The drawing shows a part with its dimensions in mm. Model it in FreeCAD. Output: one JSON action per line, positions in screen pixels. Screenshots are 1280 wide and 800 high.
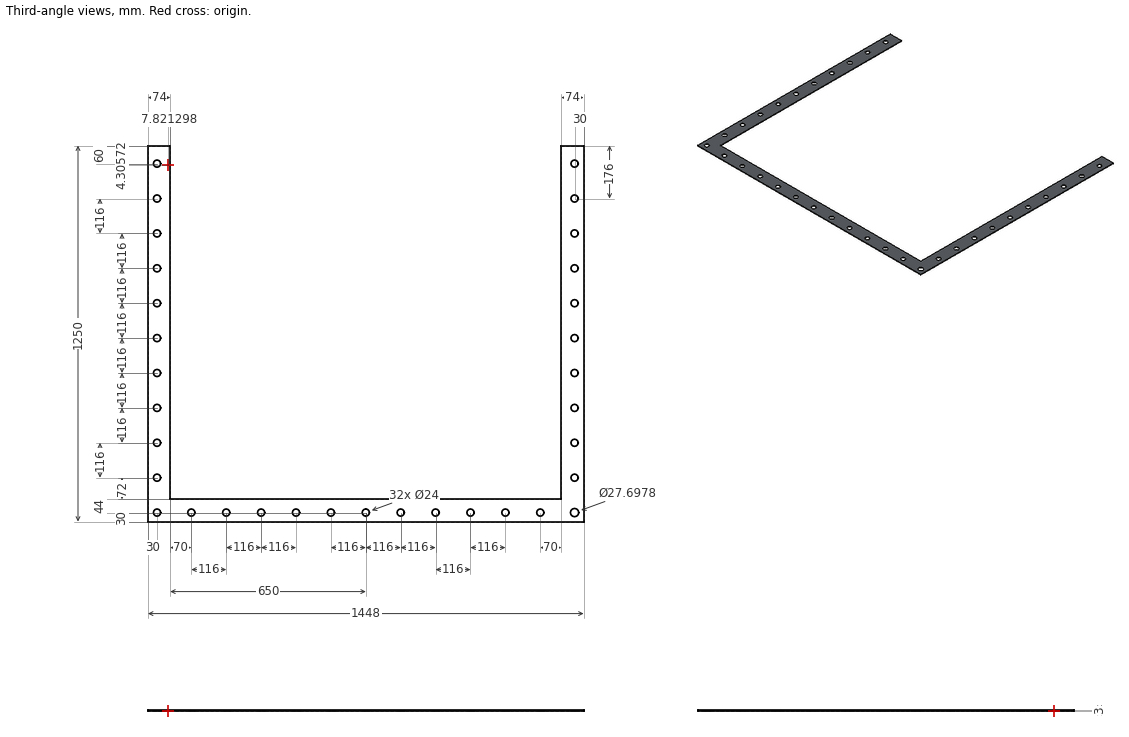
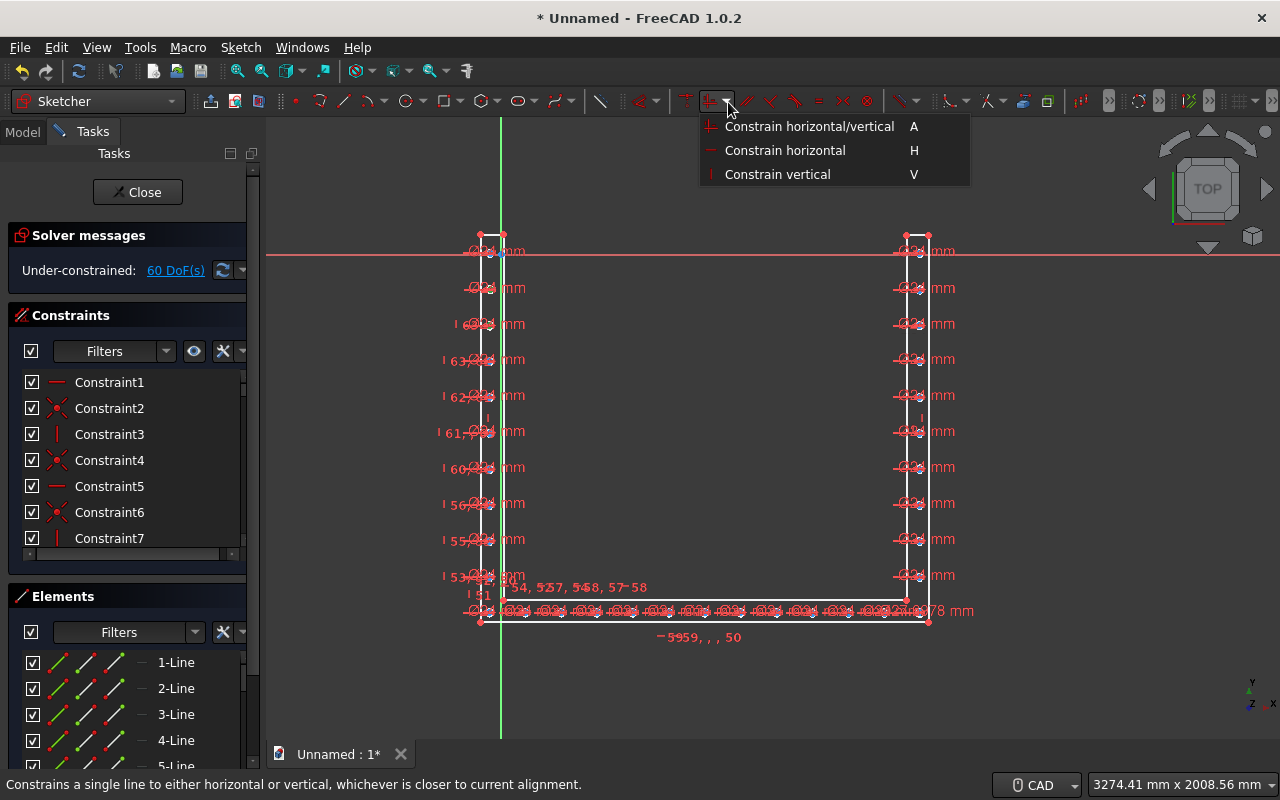
{"action": "left_click", "coordinate": [835, 174]}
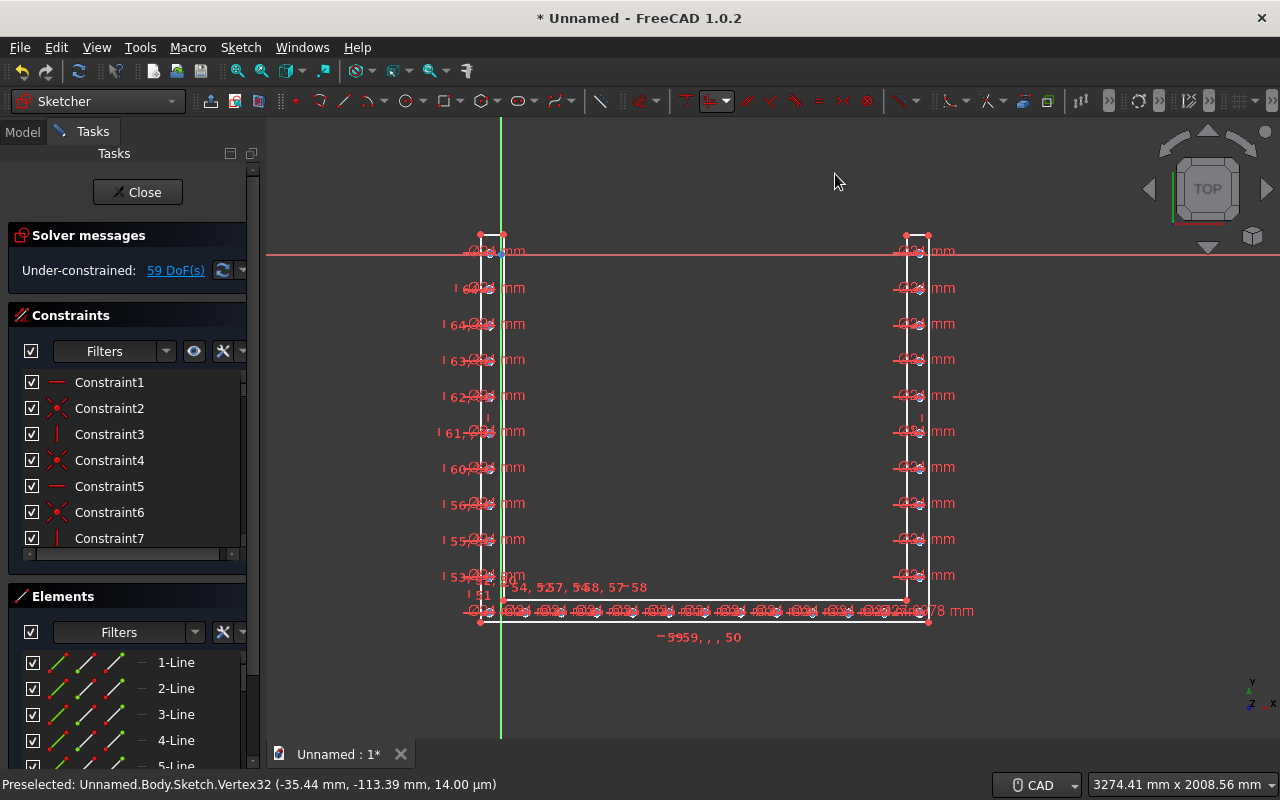
{"action": "left_click", "coordinate": [490, 290]}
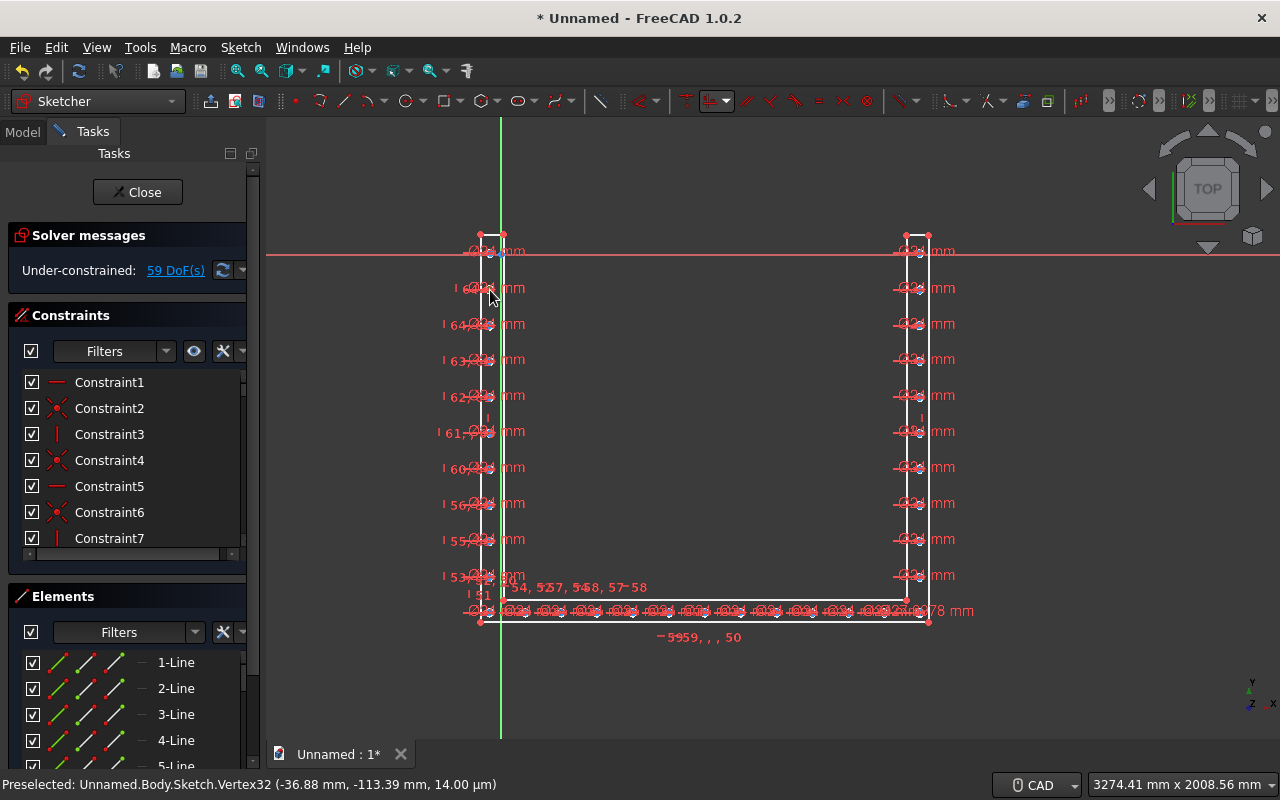
{"action": "left_click", "coordinate": [490, 253]}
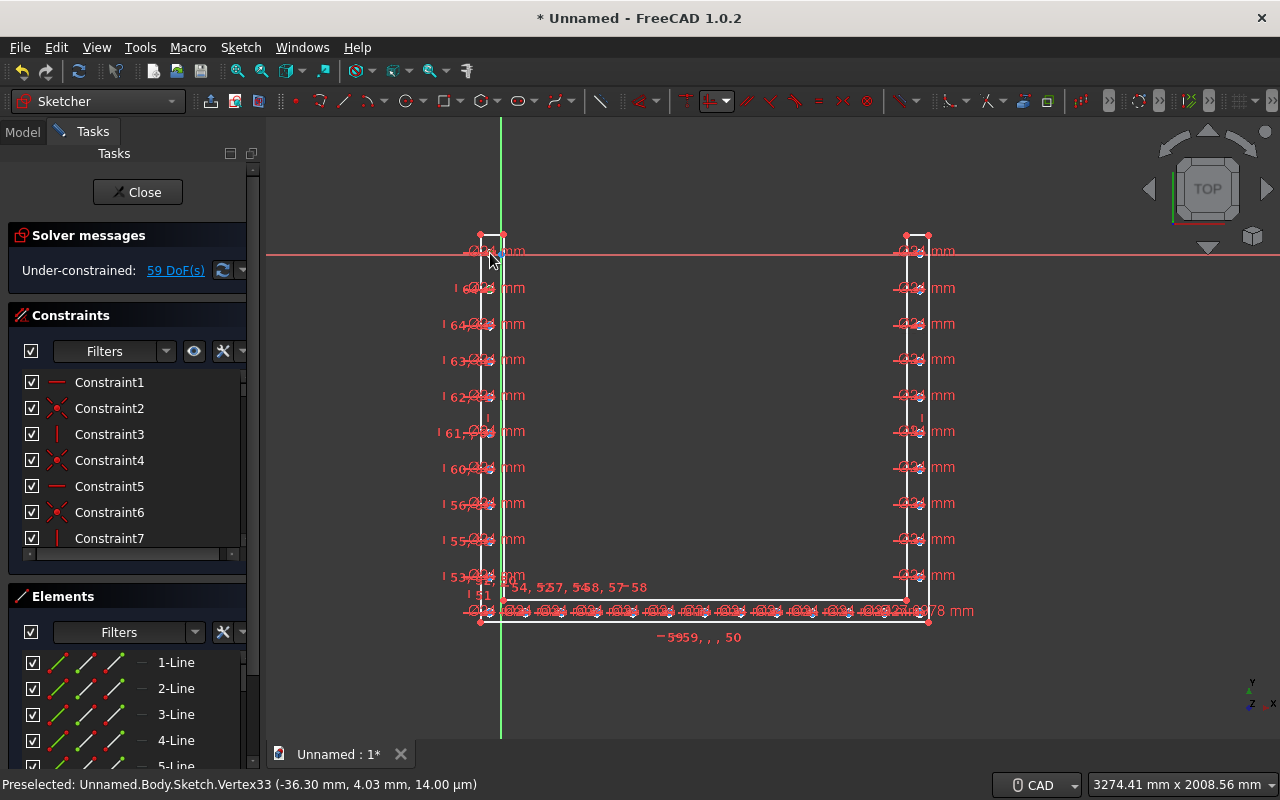
{"action": "key", "text": "v"}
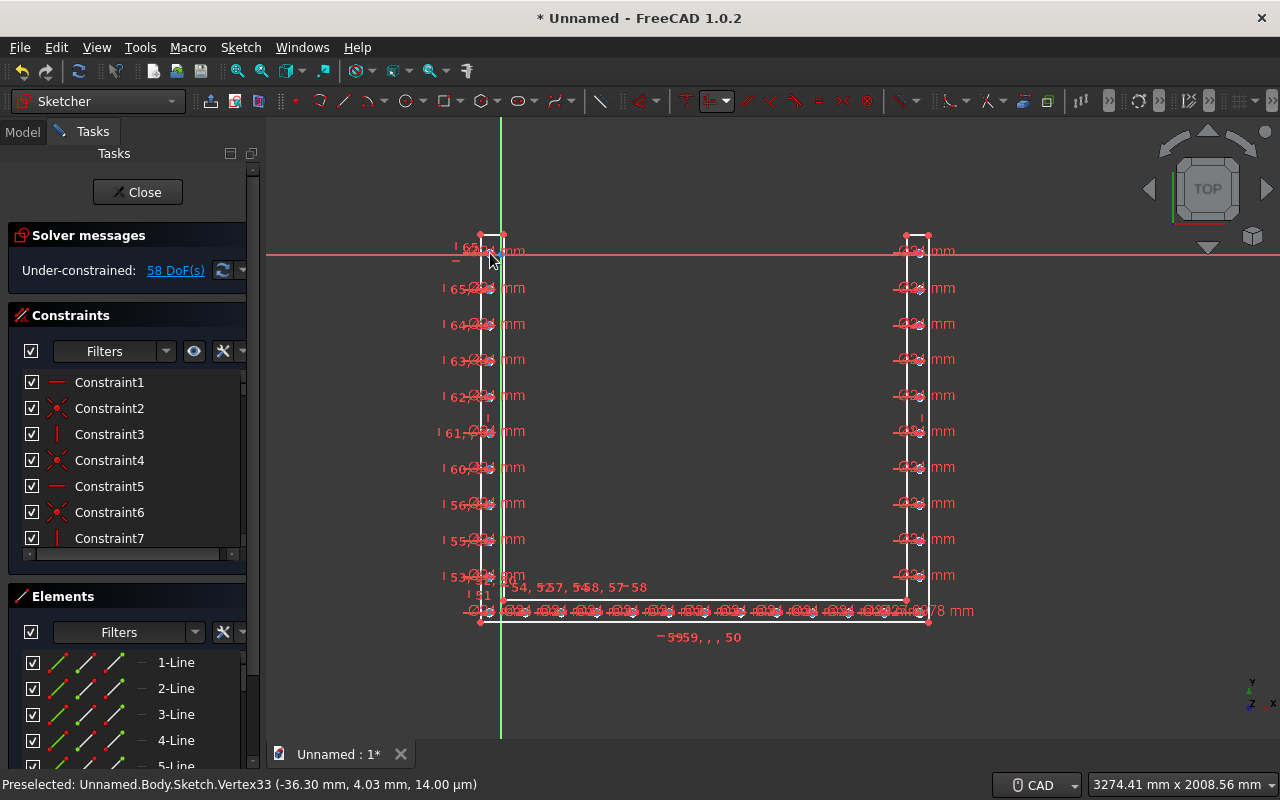
{"action": "left_click", "coordinate": [920, 290]}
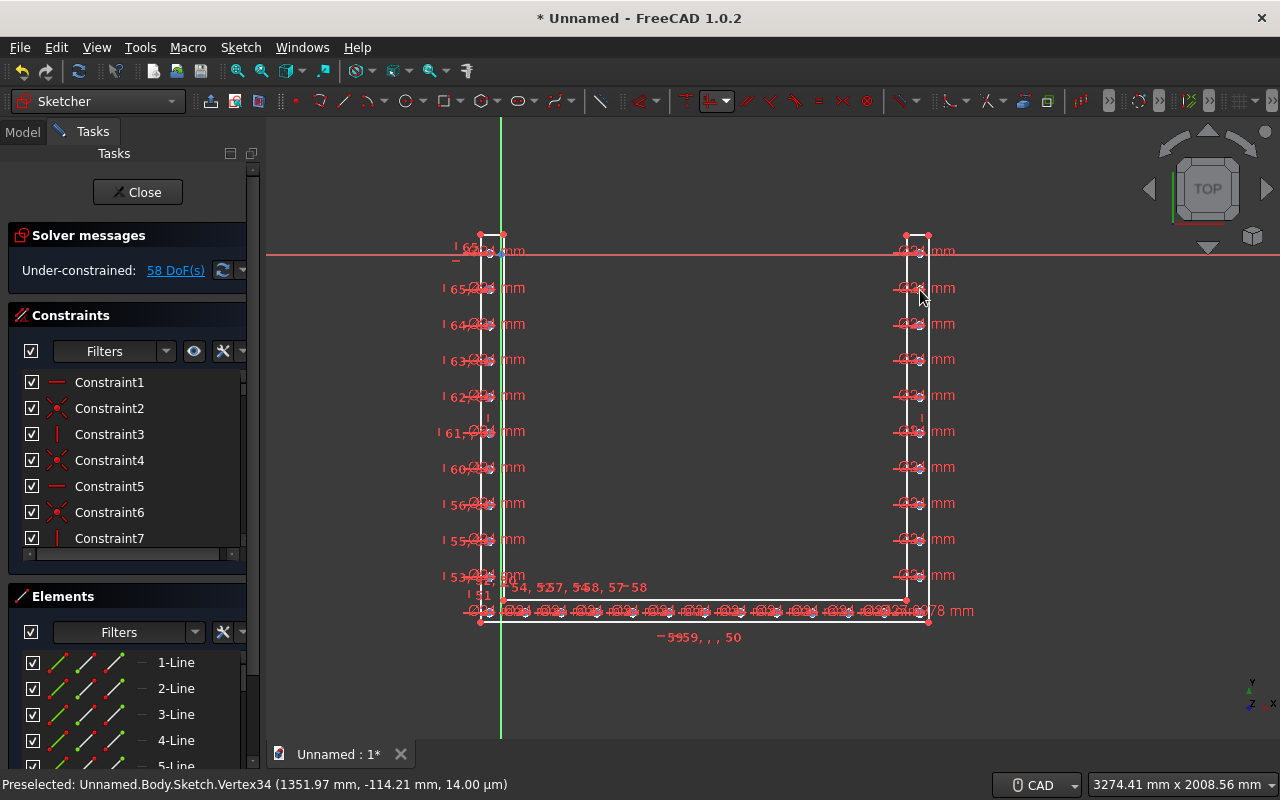
{"action": "left_click", "coordinate": [920, 253]}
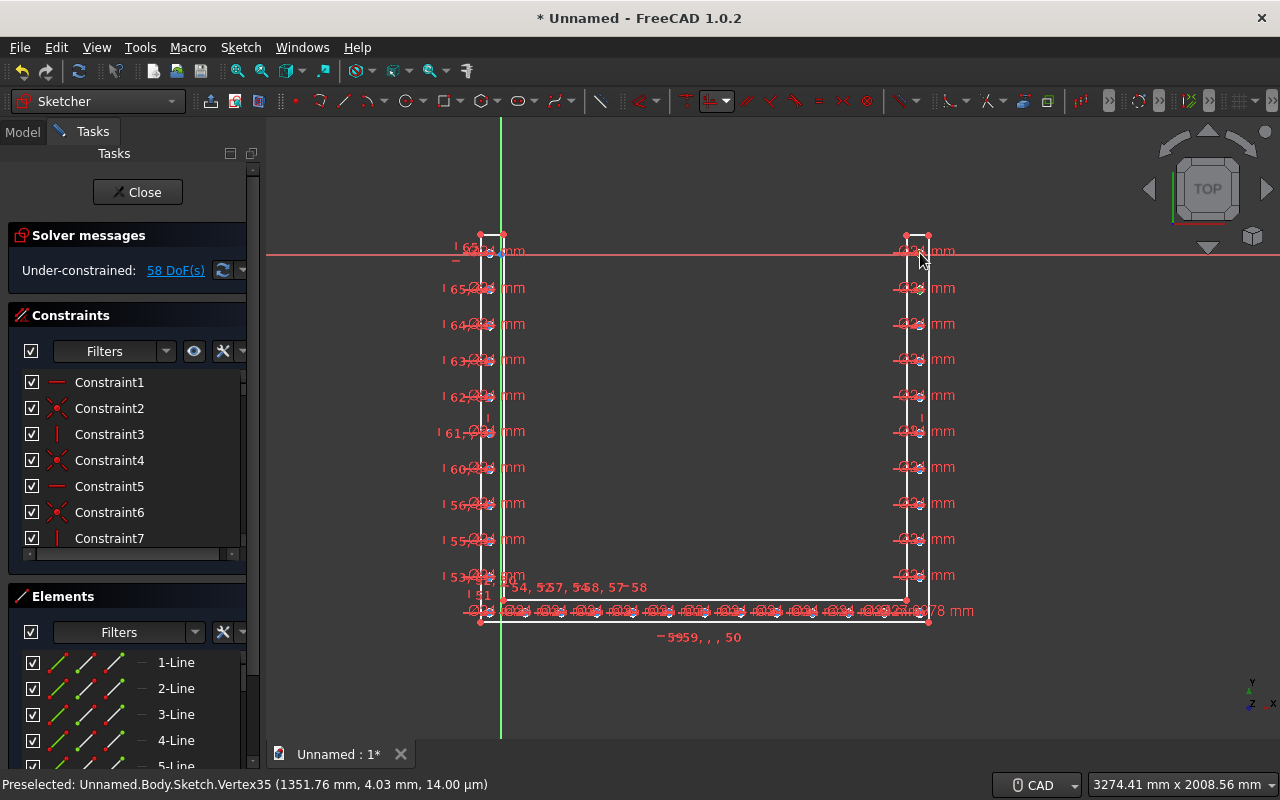
{"action": "left_click", "coordinate": [728, 102]}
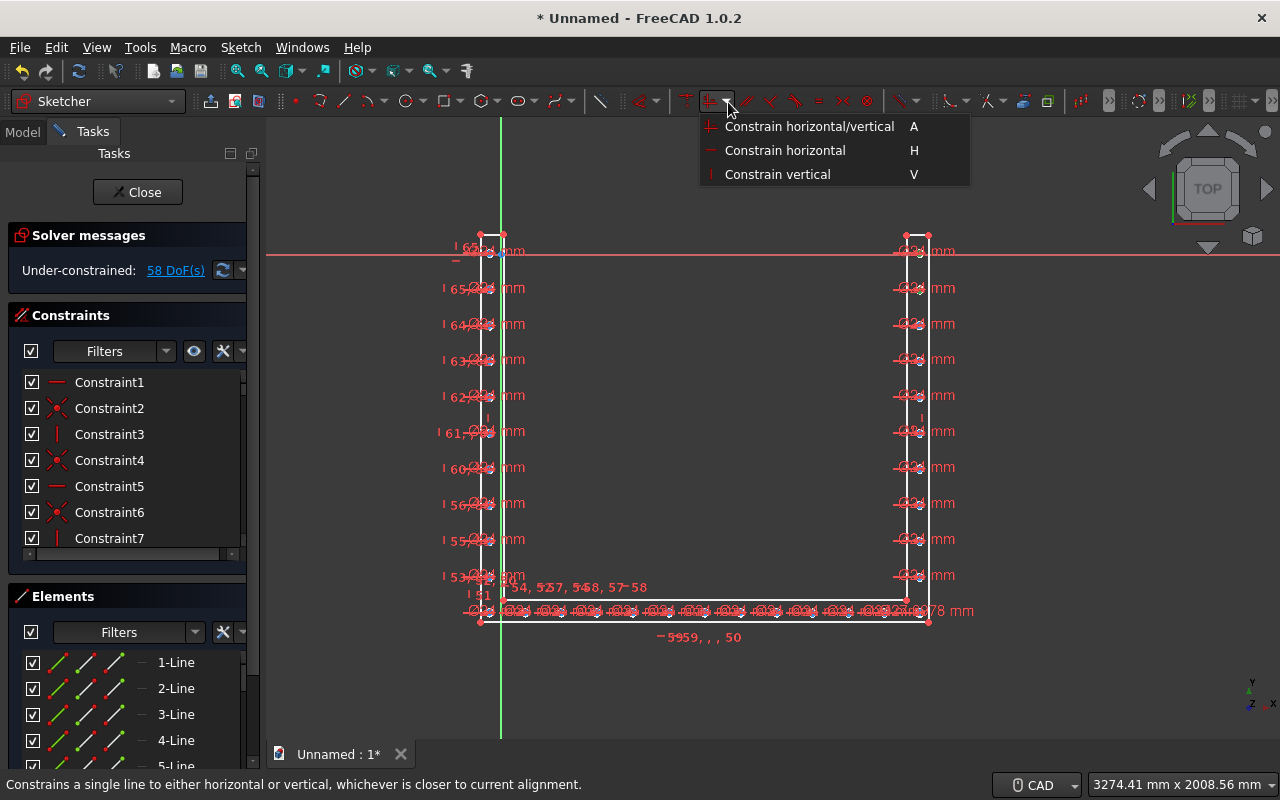
{"action": "left_click", "coordinate": [835, 174]}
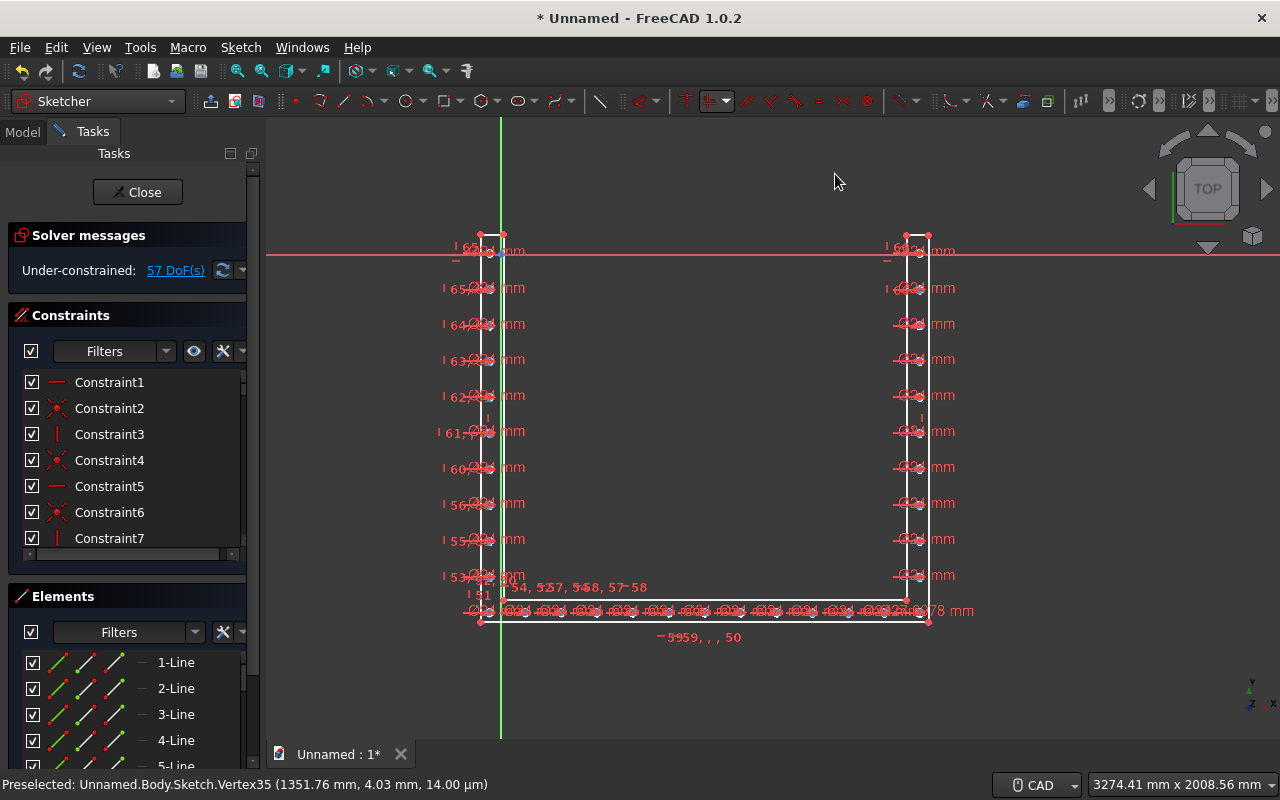
{"action": "left_click", "coordinate": [705, 613]}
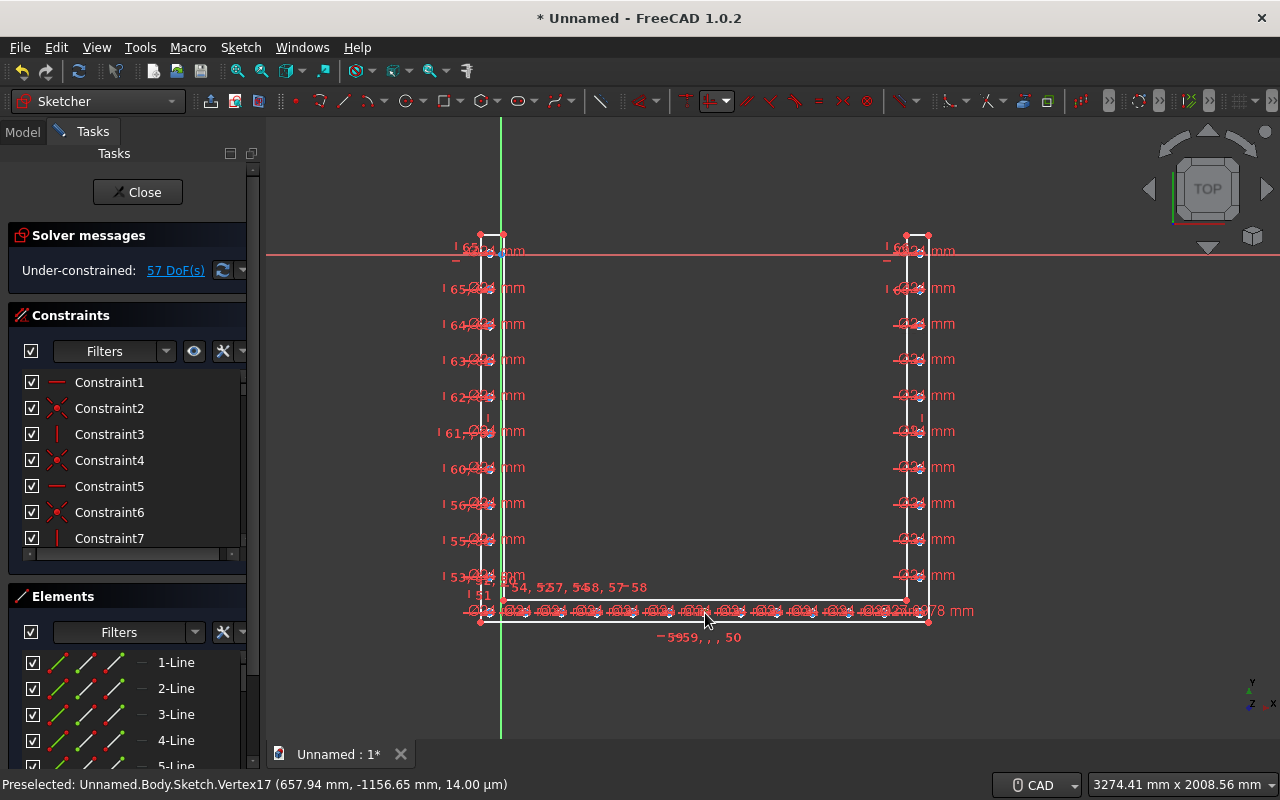
{"action": "left_click", "coordinate": [741, 613]}